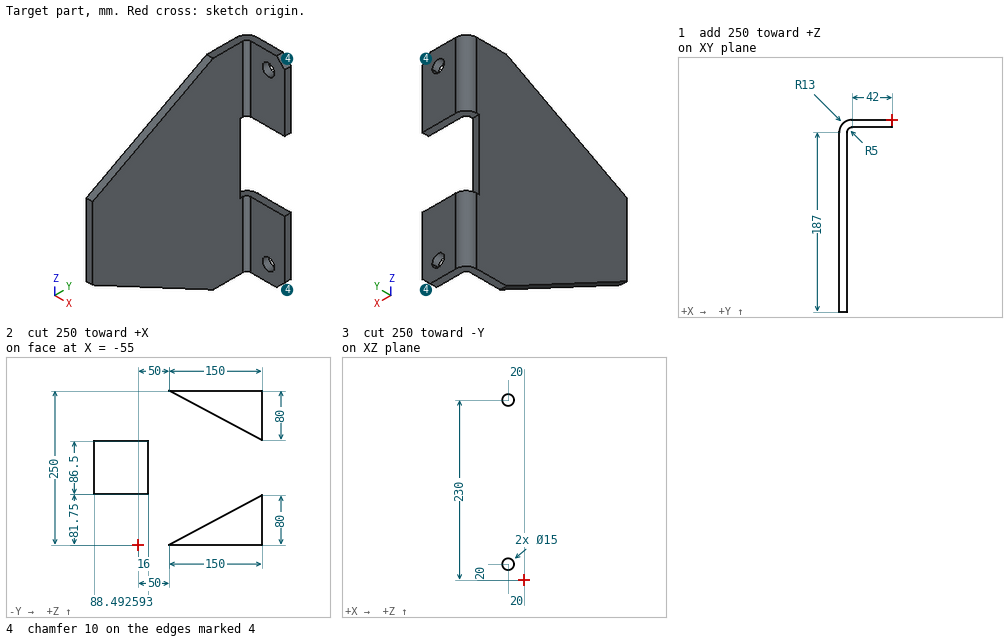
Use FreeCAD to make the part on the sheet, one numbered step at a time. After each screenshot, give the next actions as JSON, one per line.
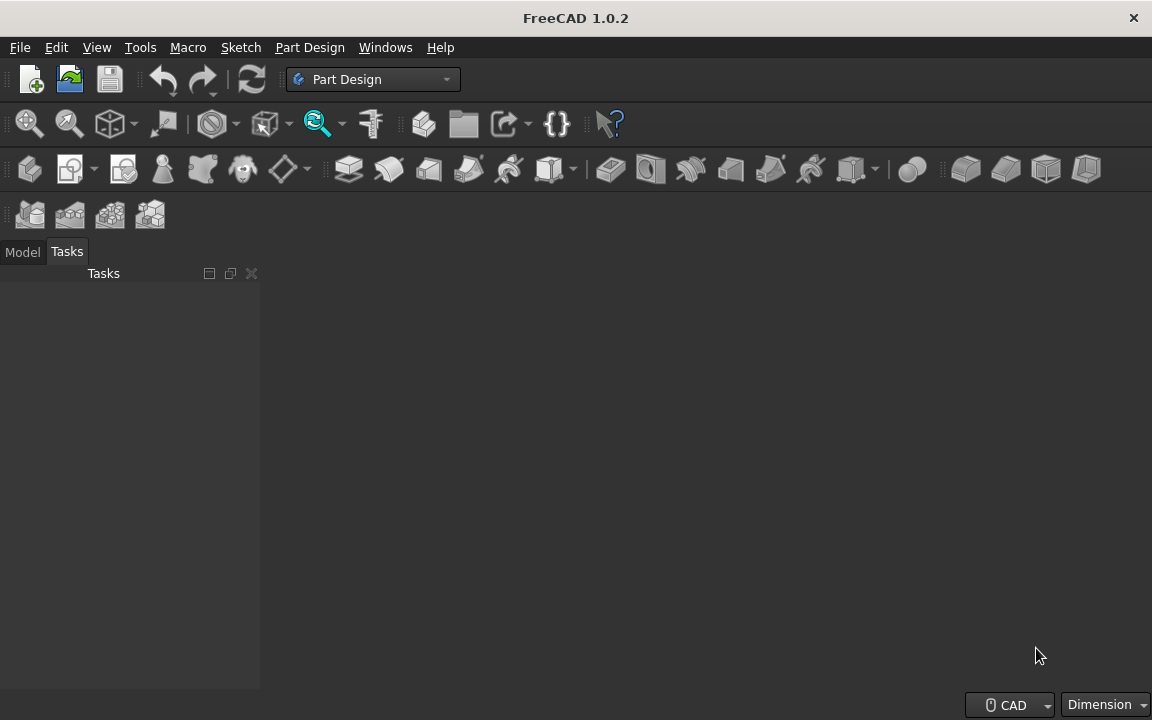
{"action": "left_click", "coordinate": [30, 80]}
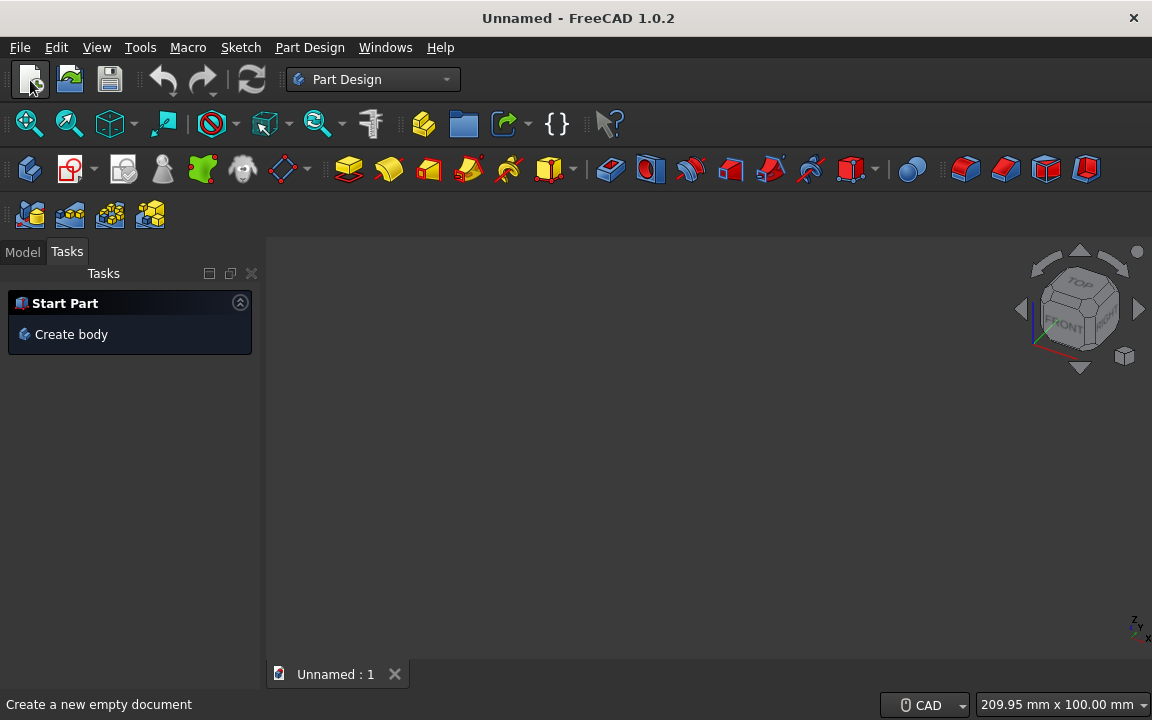
{"action": "left_click", "coordinate": [70, 170]}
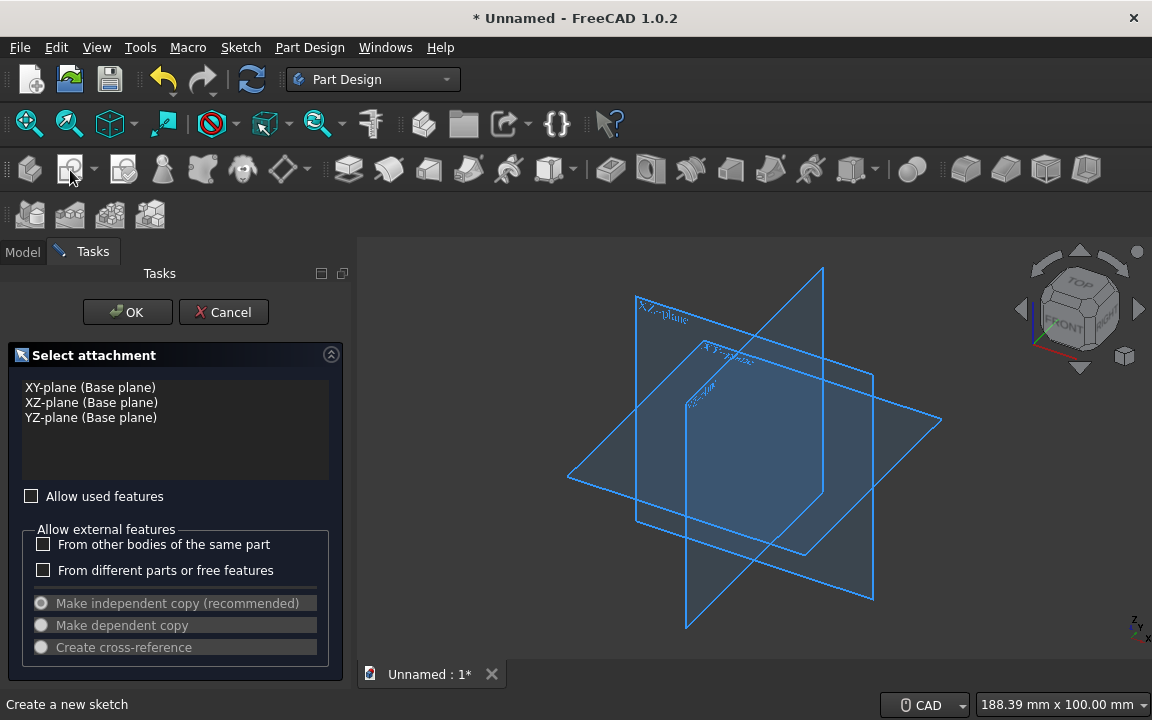
{"action": "left_click", "coordinate": [82, 388]}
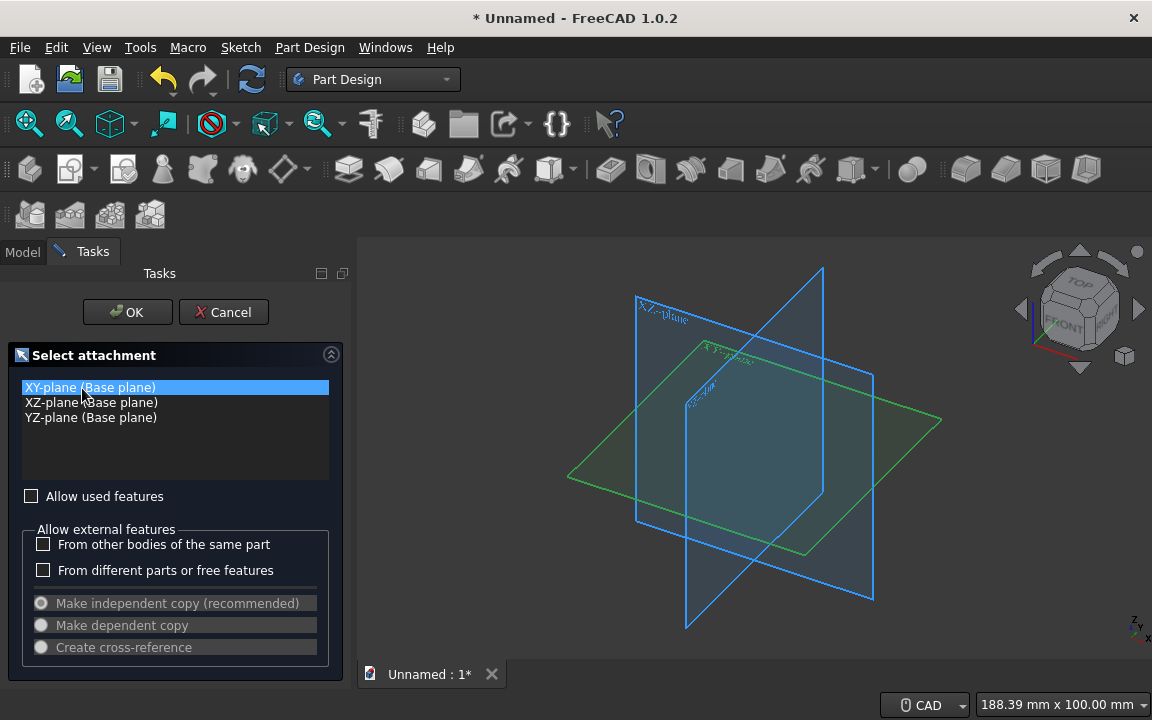
{"action": "left_click", "coordinate": [128, 312]}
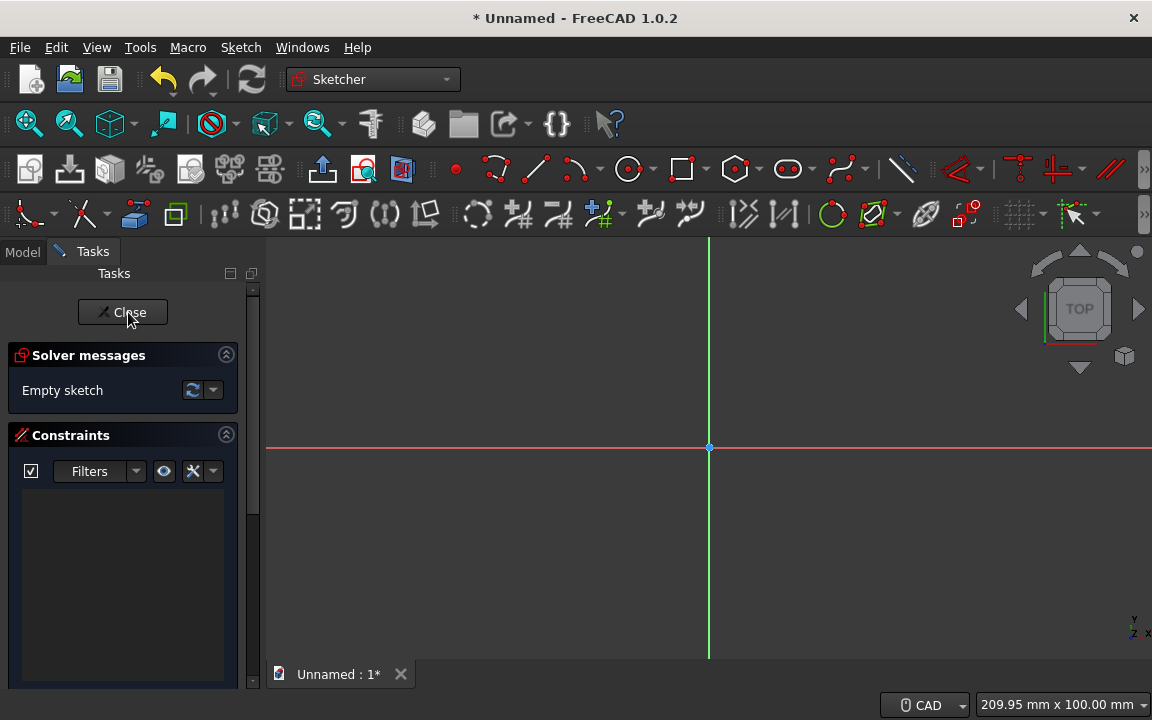
{"action": "scroll", "coordinate": [661, 266], "scroll_direction": "down", "scroll_amount": 6}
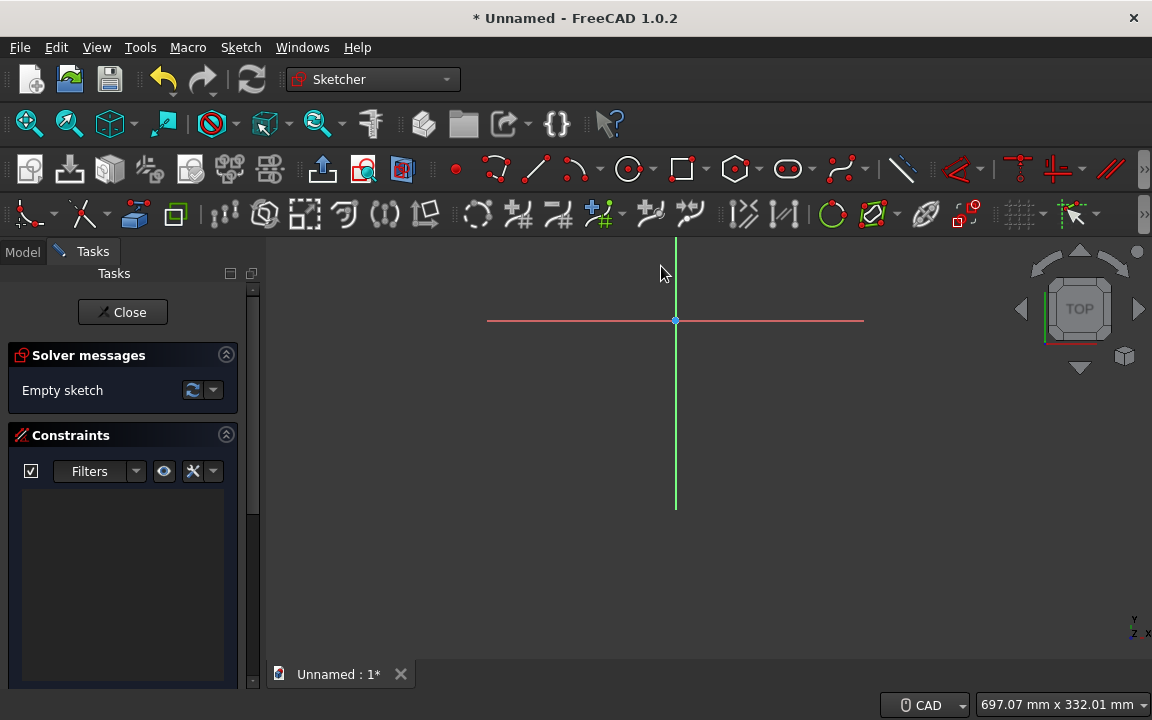
{"action": "key", "text": "g m"}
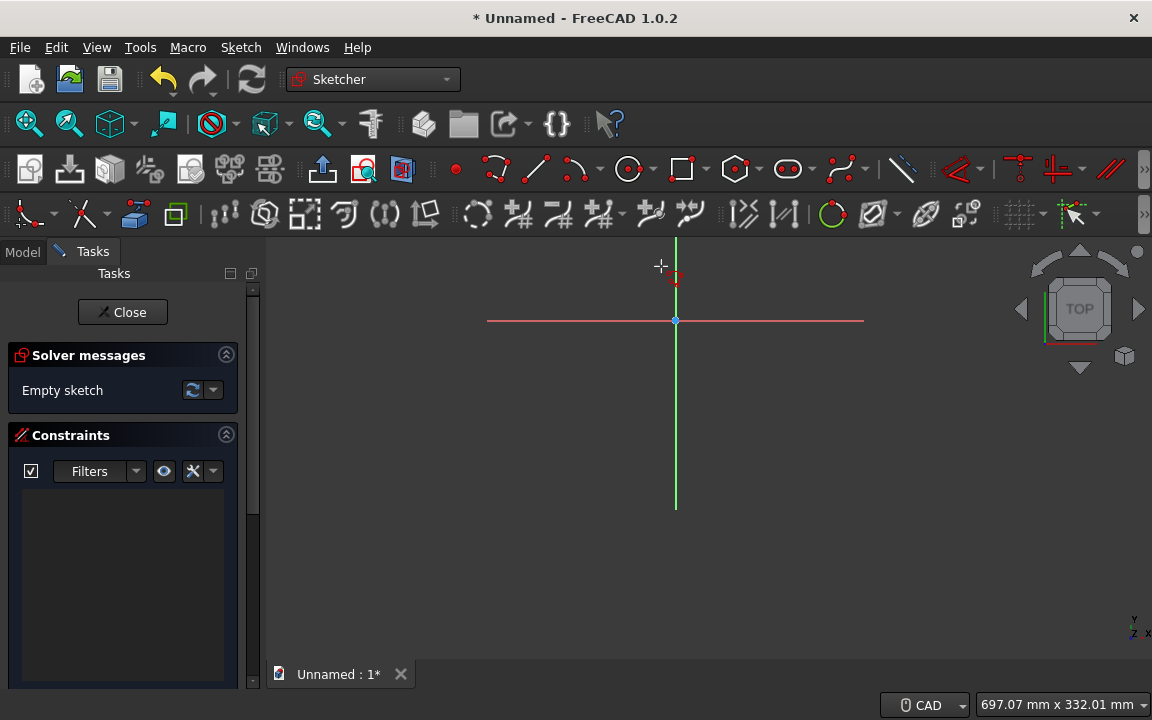
{"action": "left_click", "coordinate": [606, 337]}
{"action": "left_click", "coordinate": [606, 575]}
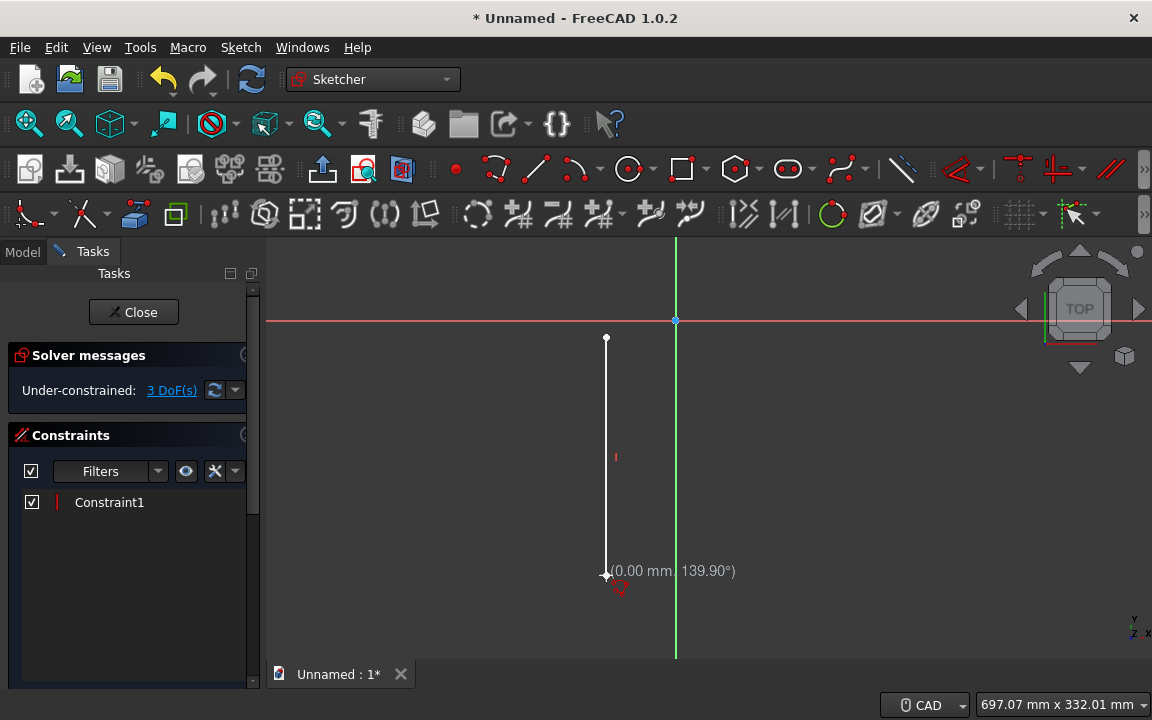
{"action": "scroll", "coordinate": [616, 575], "scroll_direction": "up", "scroll_amount": 3}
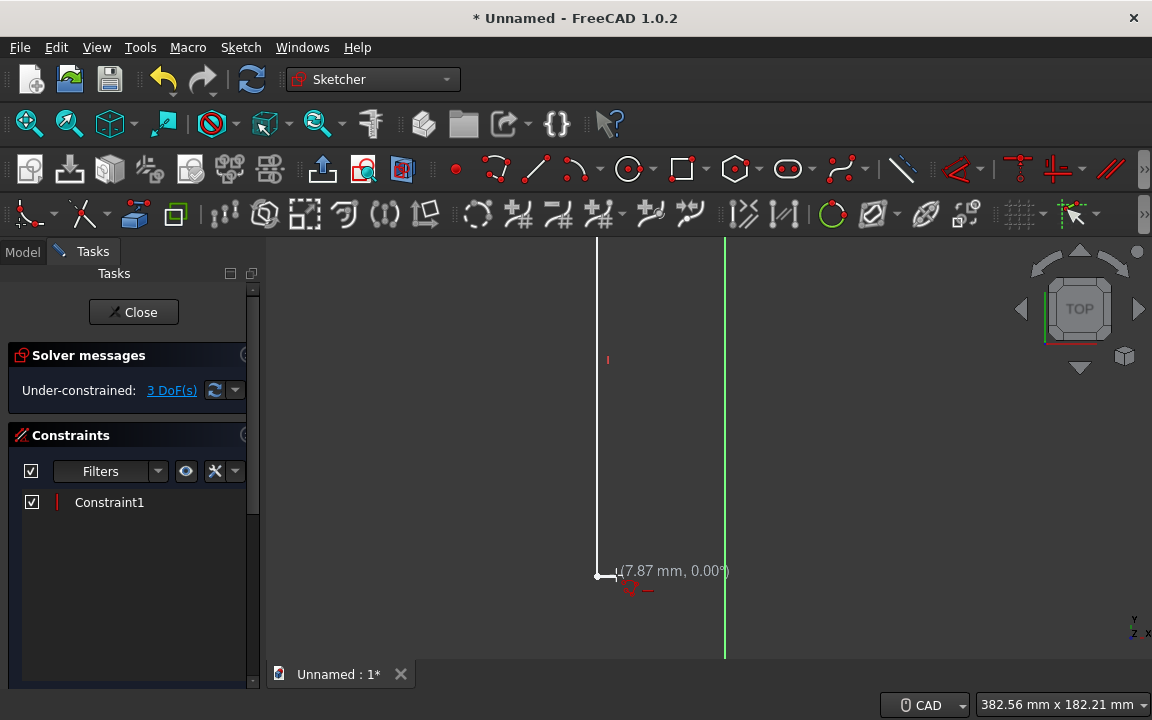
{"action": "left_click", "coordinate": [616, 574]}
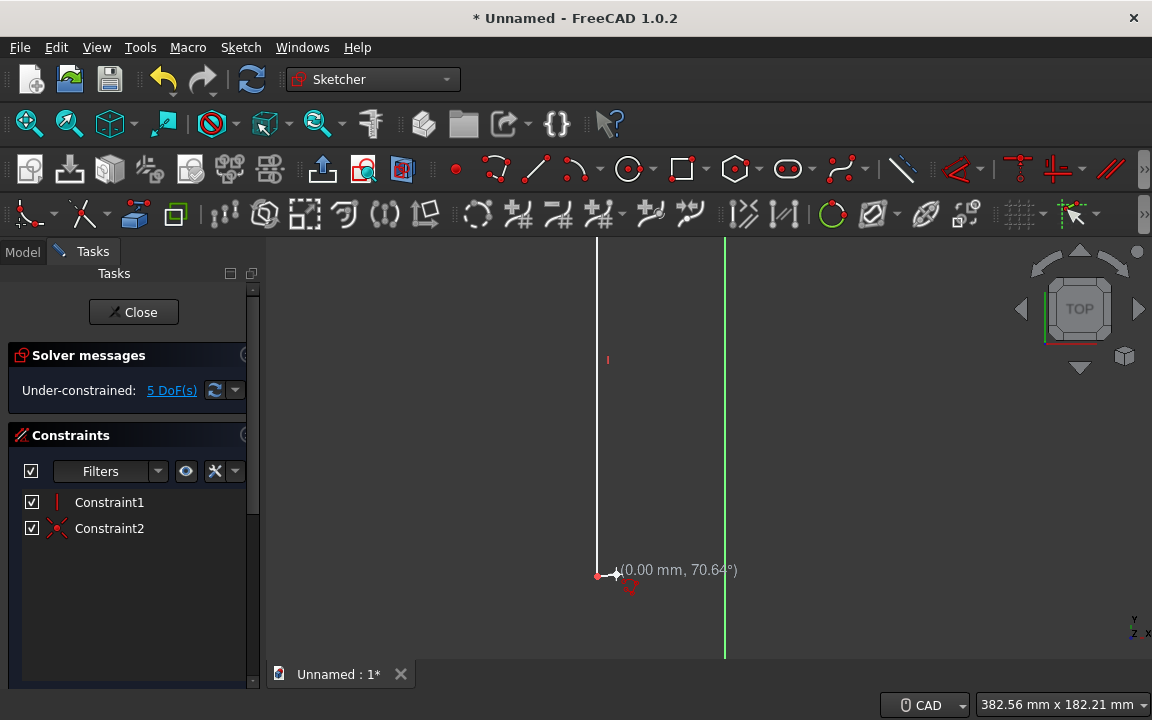
{"action": "scroll", "coordinate": [616, 576], "scroll_direction": "down", "scroll_amount": 3}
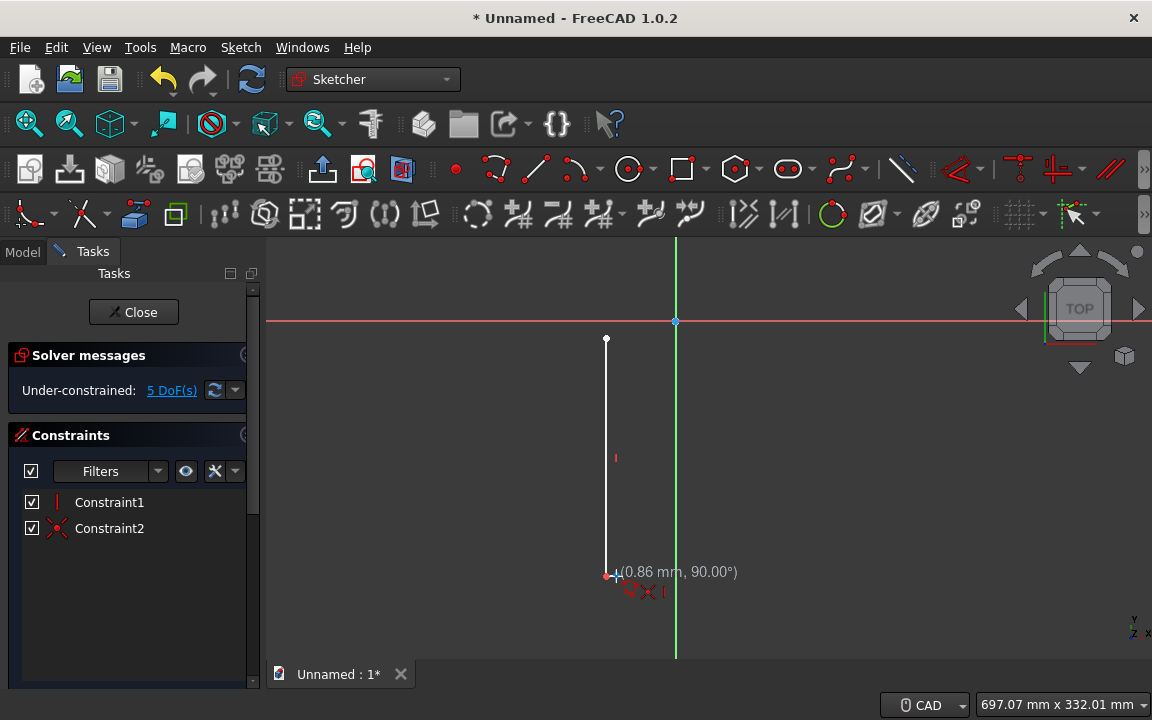
{"action": "scroll", "coordinate": [616, 338], "scroll_direction": "up", "scroll_amount": 3}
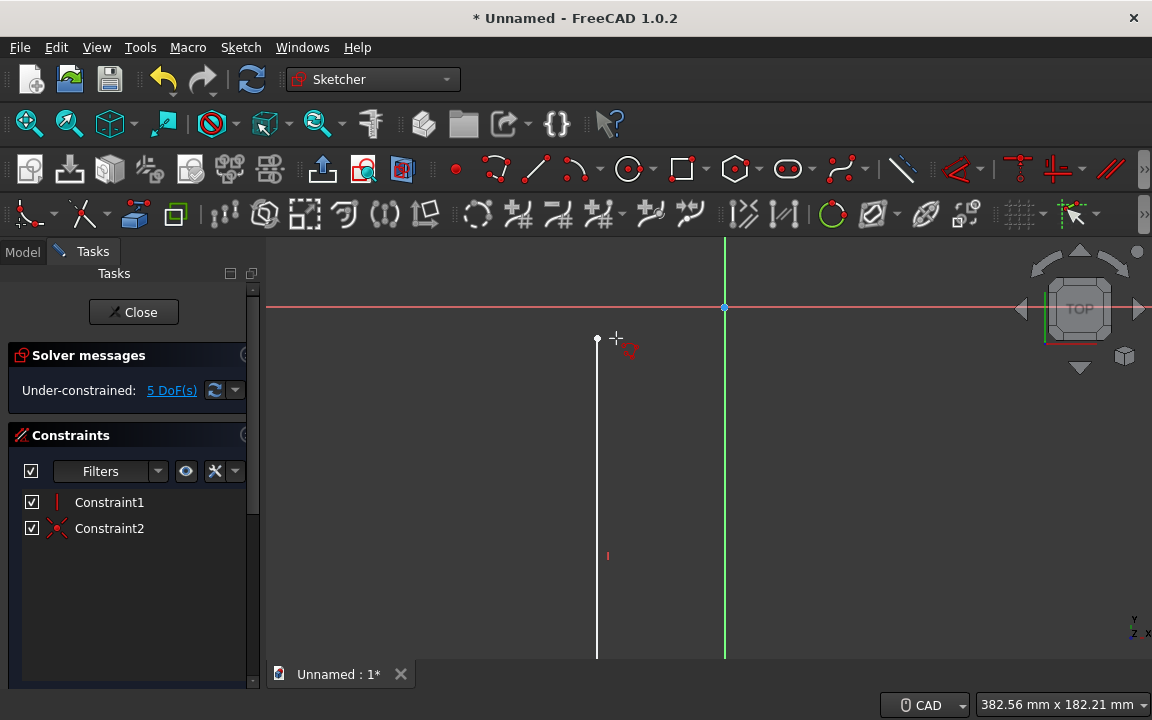
{"action": "left_click", "coordinate": [616, 338]}
{"action": "right_click", "coordinate": [616, 338]}